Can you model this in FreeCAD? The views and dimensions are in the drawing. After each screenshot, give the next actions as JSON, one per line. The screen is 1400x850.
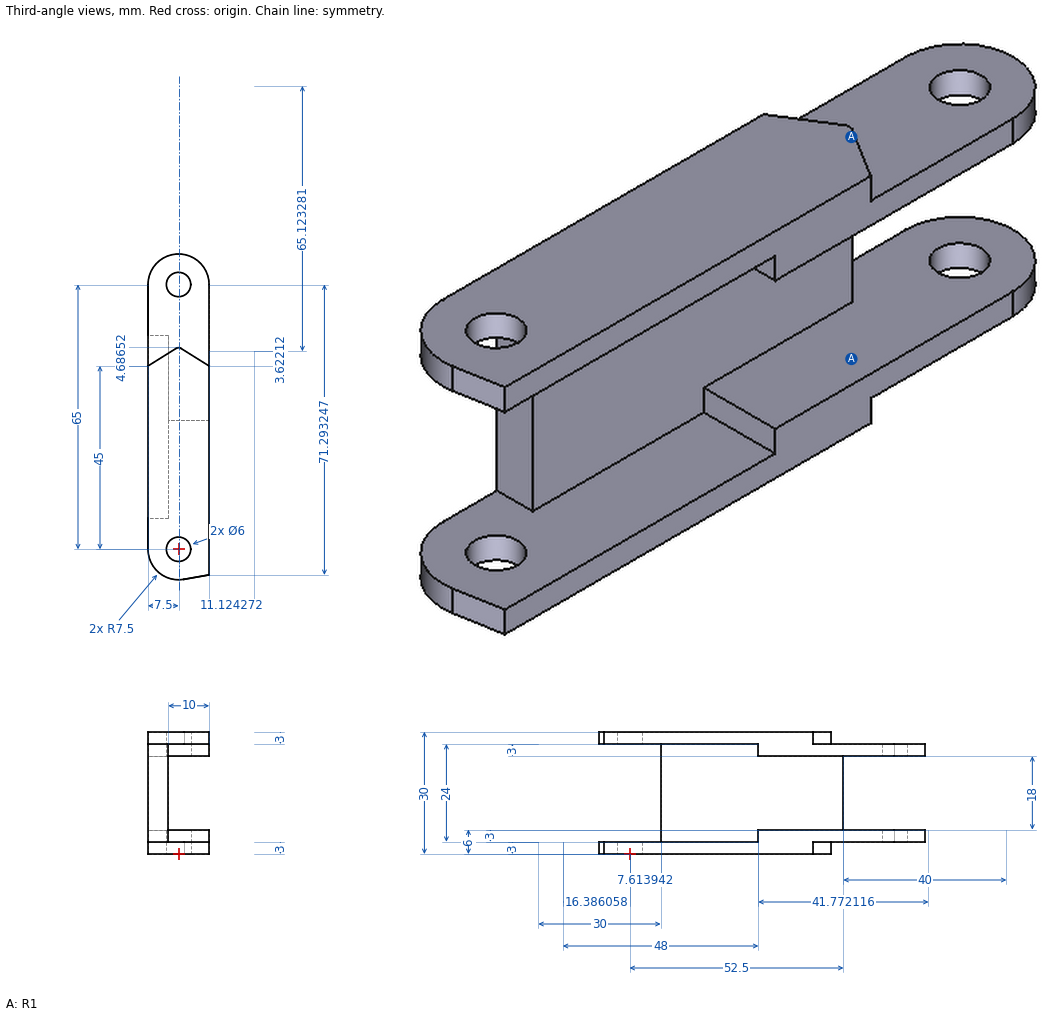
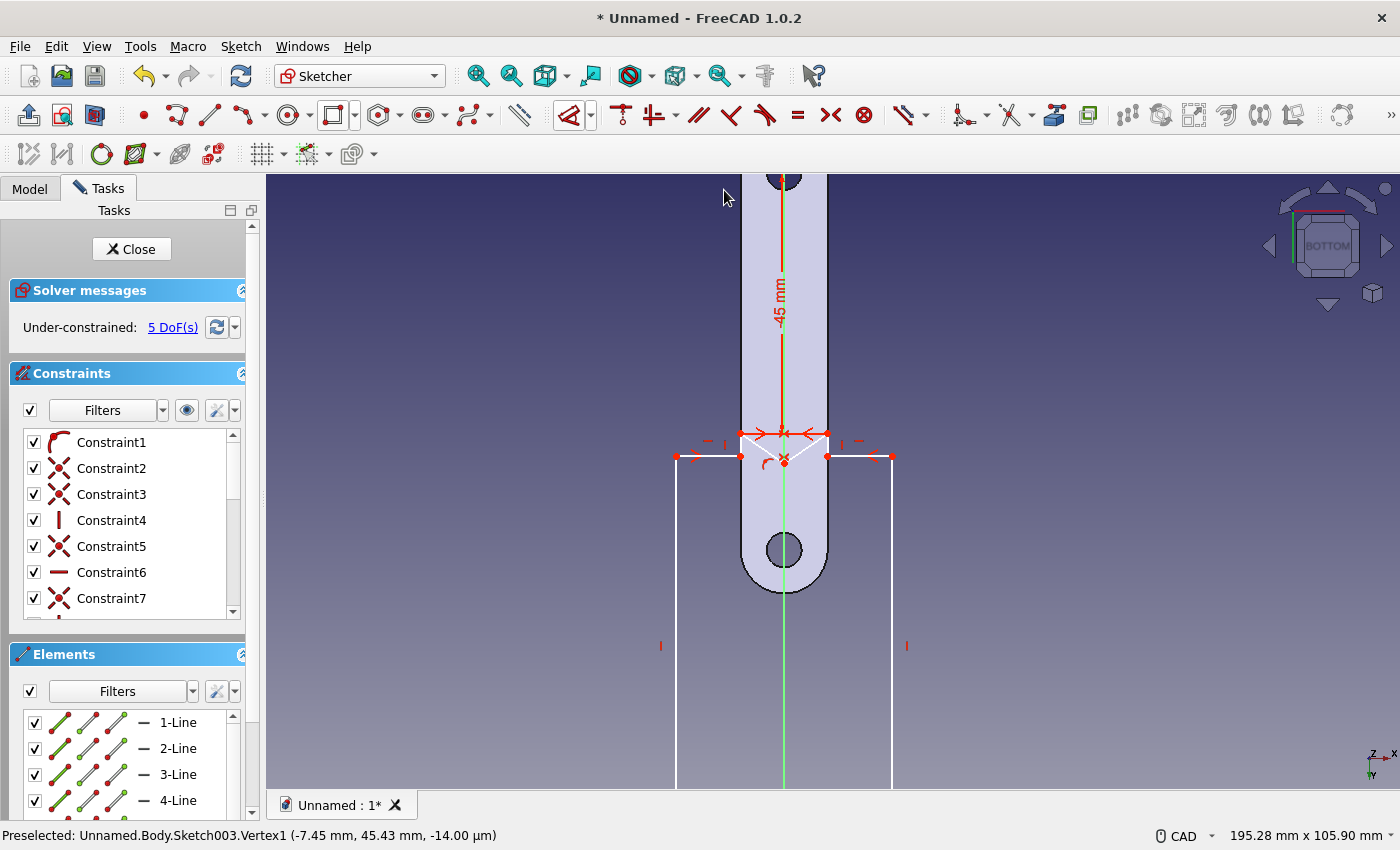
{"action": "left_click", "coordinate": [741, 434]}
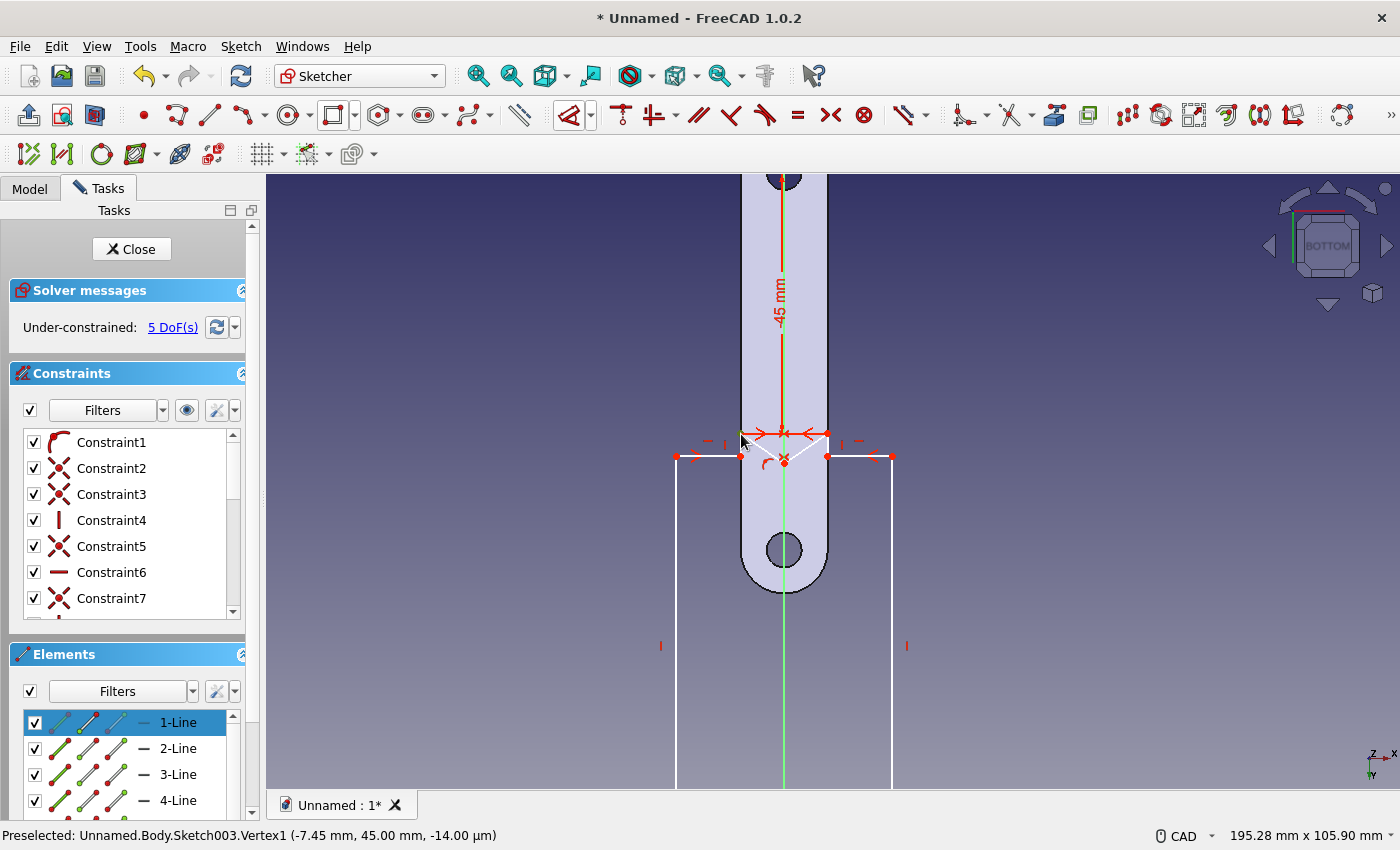
{"action": "left_click", "coordinate": [590, 116]}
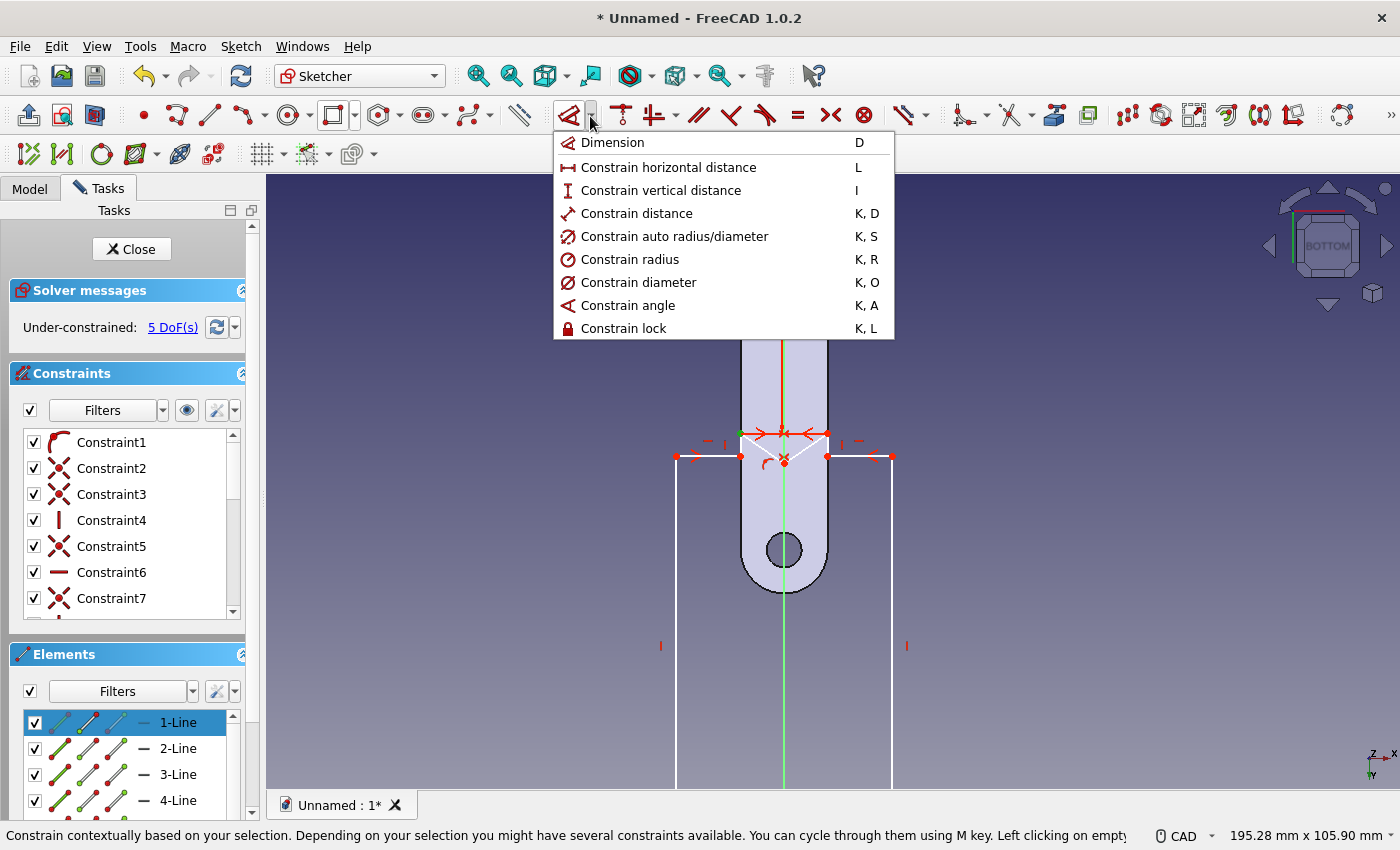
{"action": "left_click", "coordinate": [724, 168]}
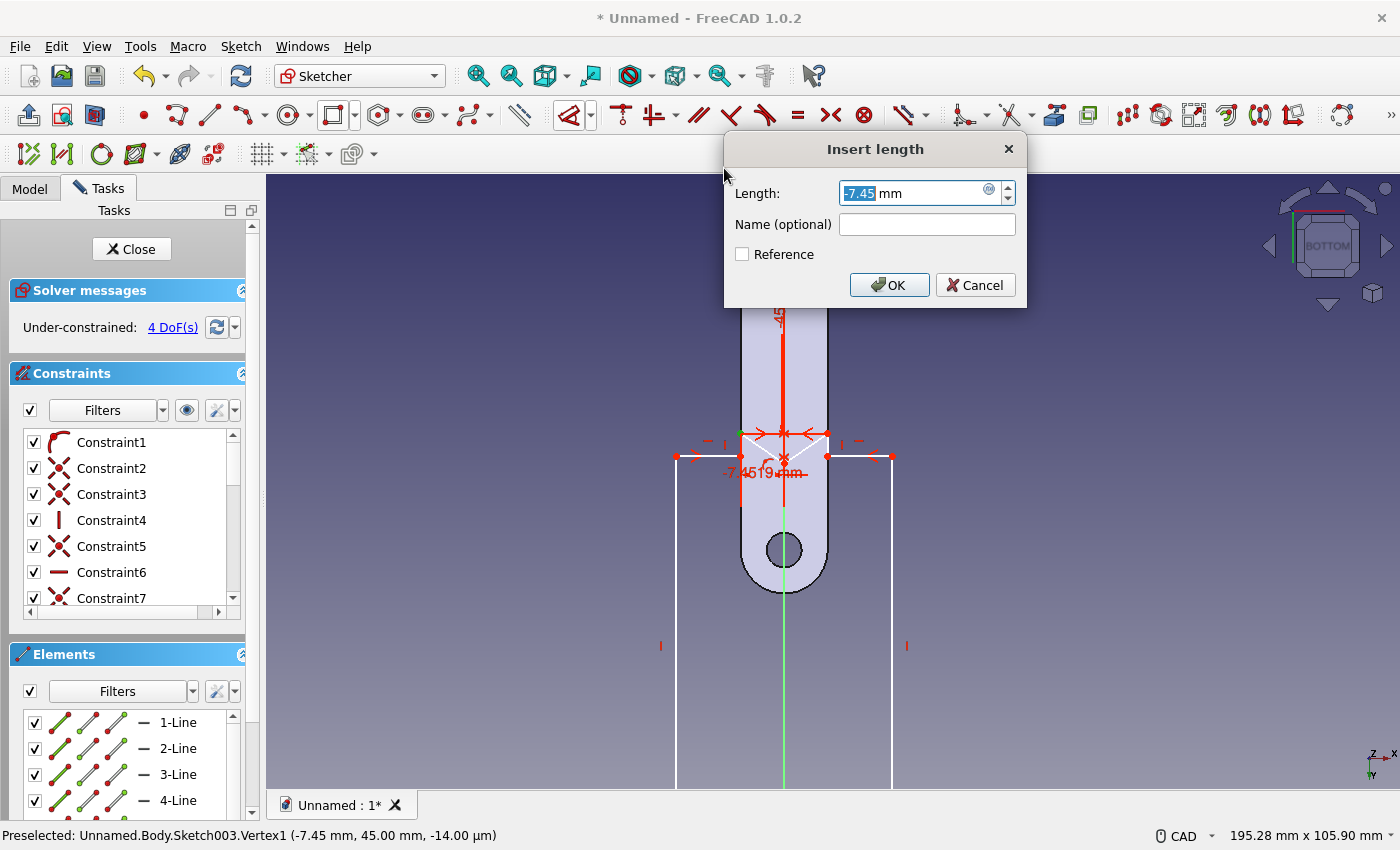
{"action": "type", "text": "-7.5"}
{"action": "key", "text": "Return"}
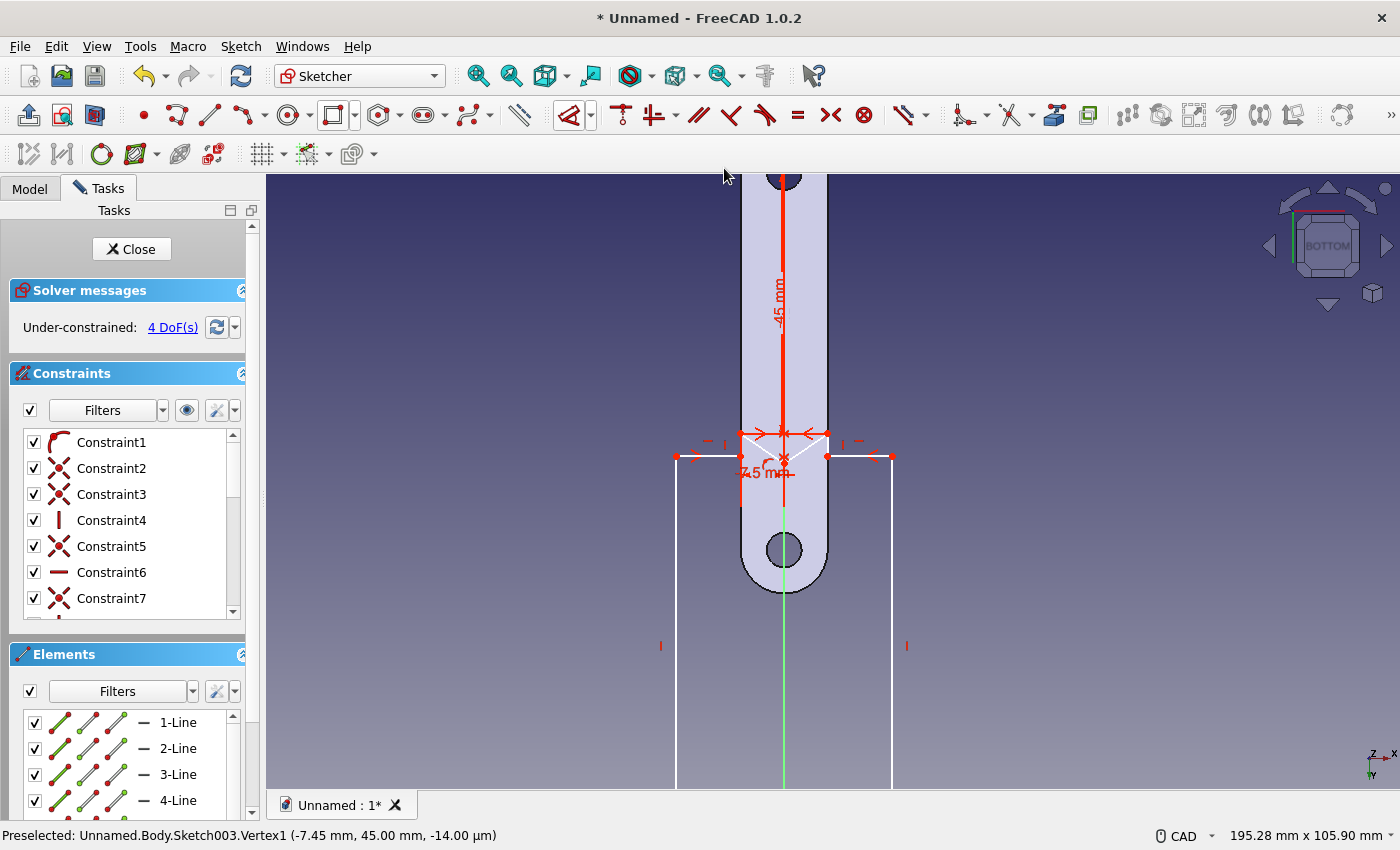
{"action": "scroll", "coordinate": [828, 445], "scroll_direction": "up", "scroll_amount": 4}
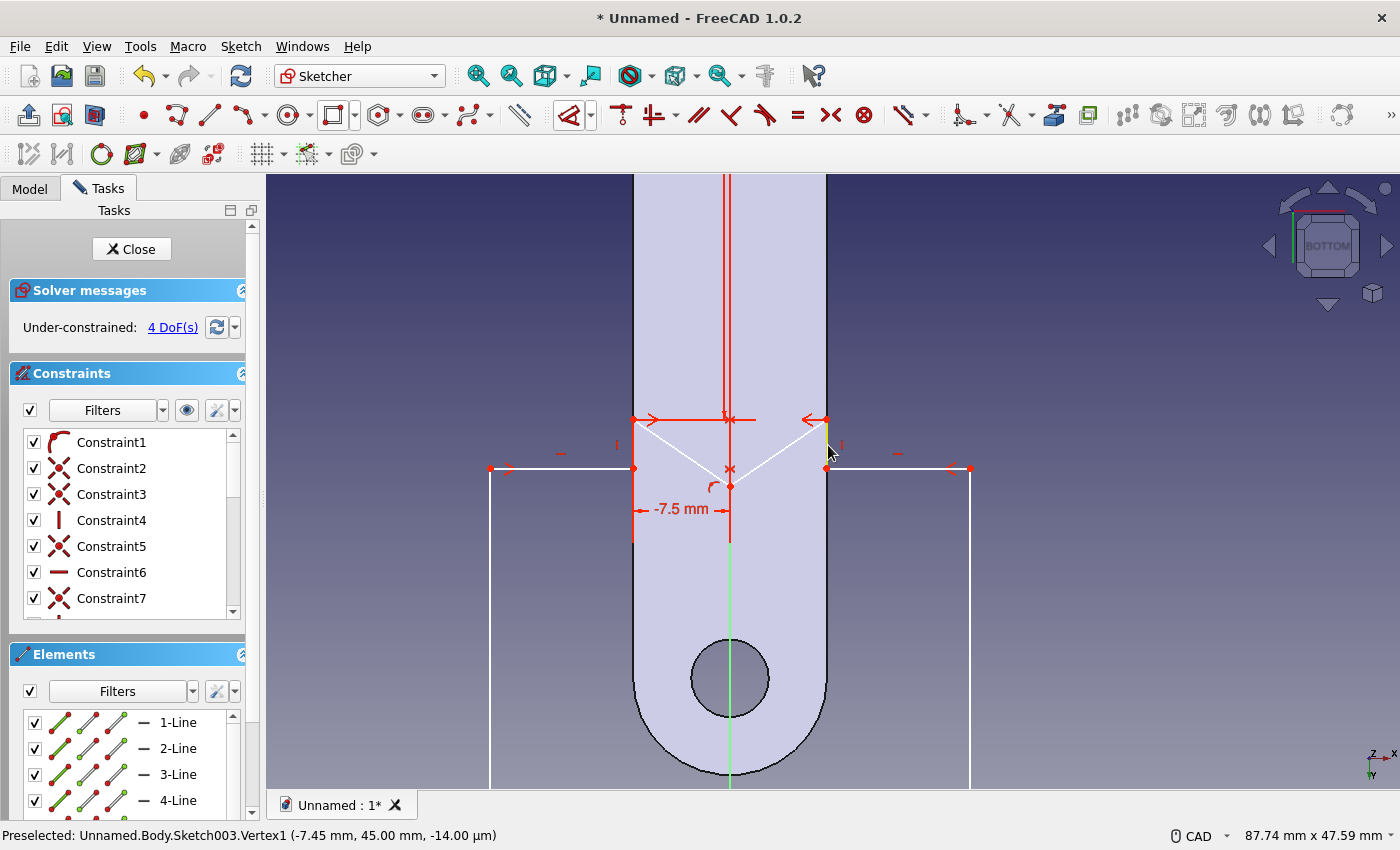
{"action": "left_click", "coordinate": [827, 444]}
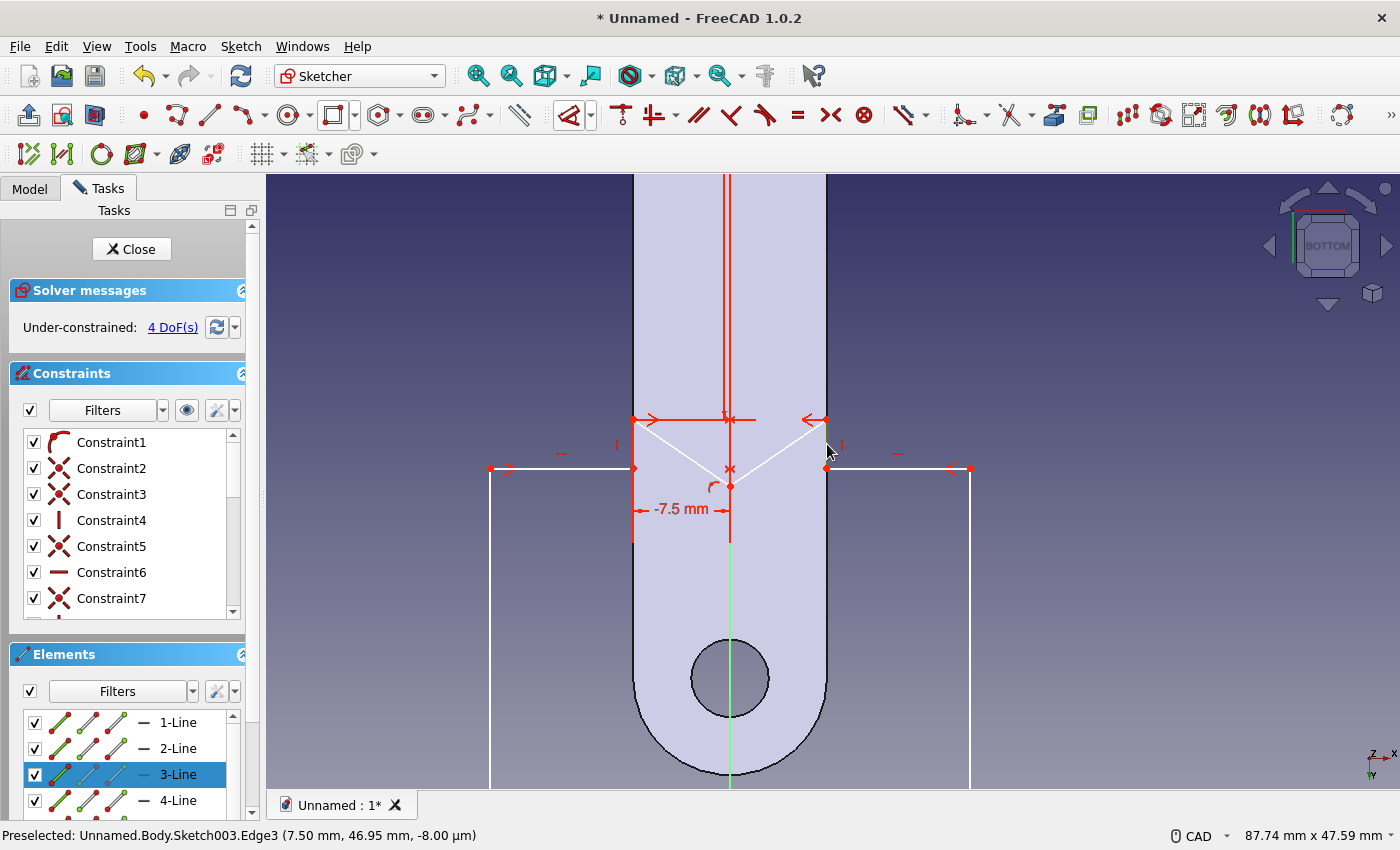
{"action": "left_click", "coordinate": [590, 116]}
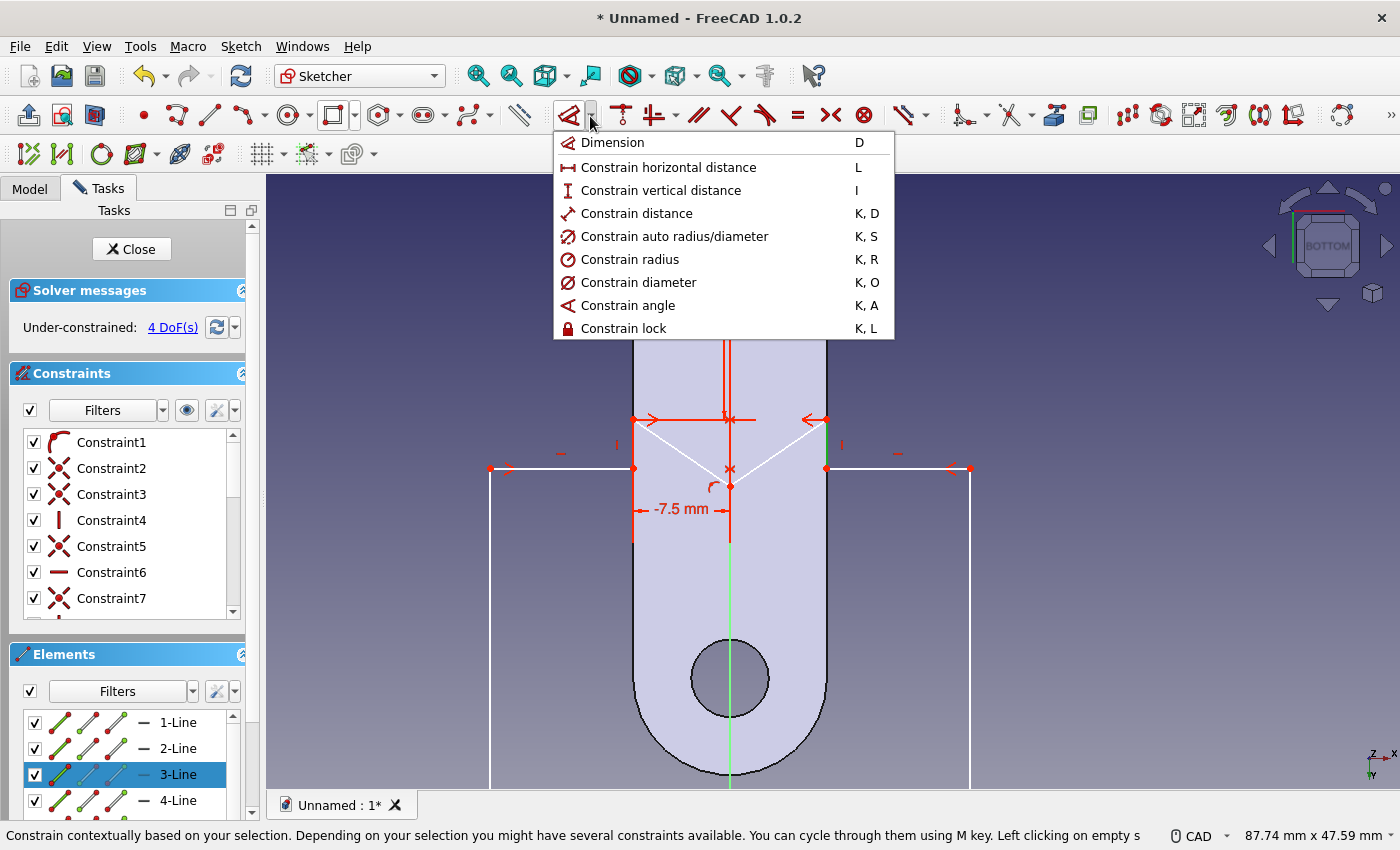
{"action": "left_click", "coordinate": [724, 190]}